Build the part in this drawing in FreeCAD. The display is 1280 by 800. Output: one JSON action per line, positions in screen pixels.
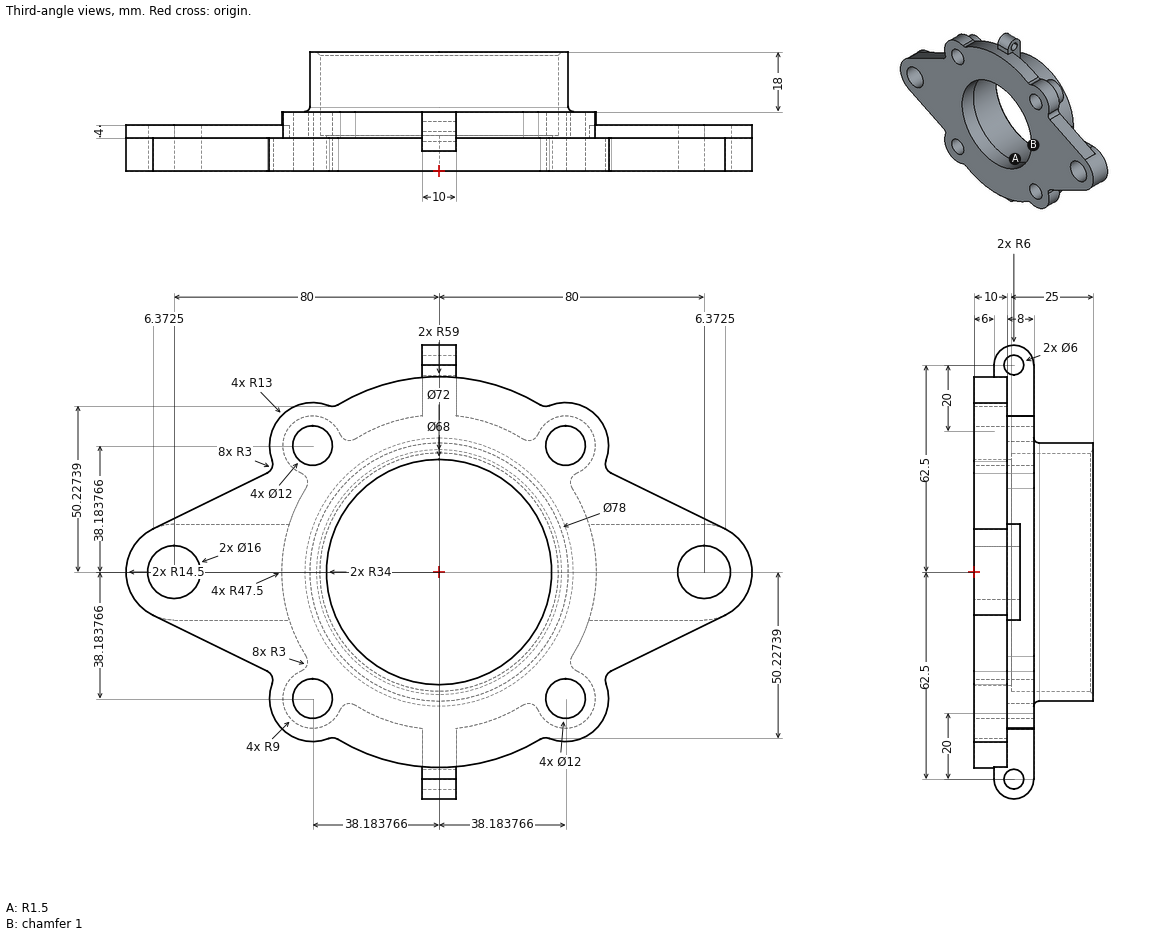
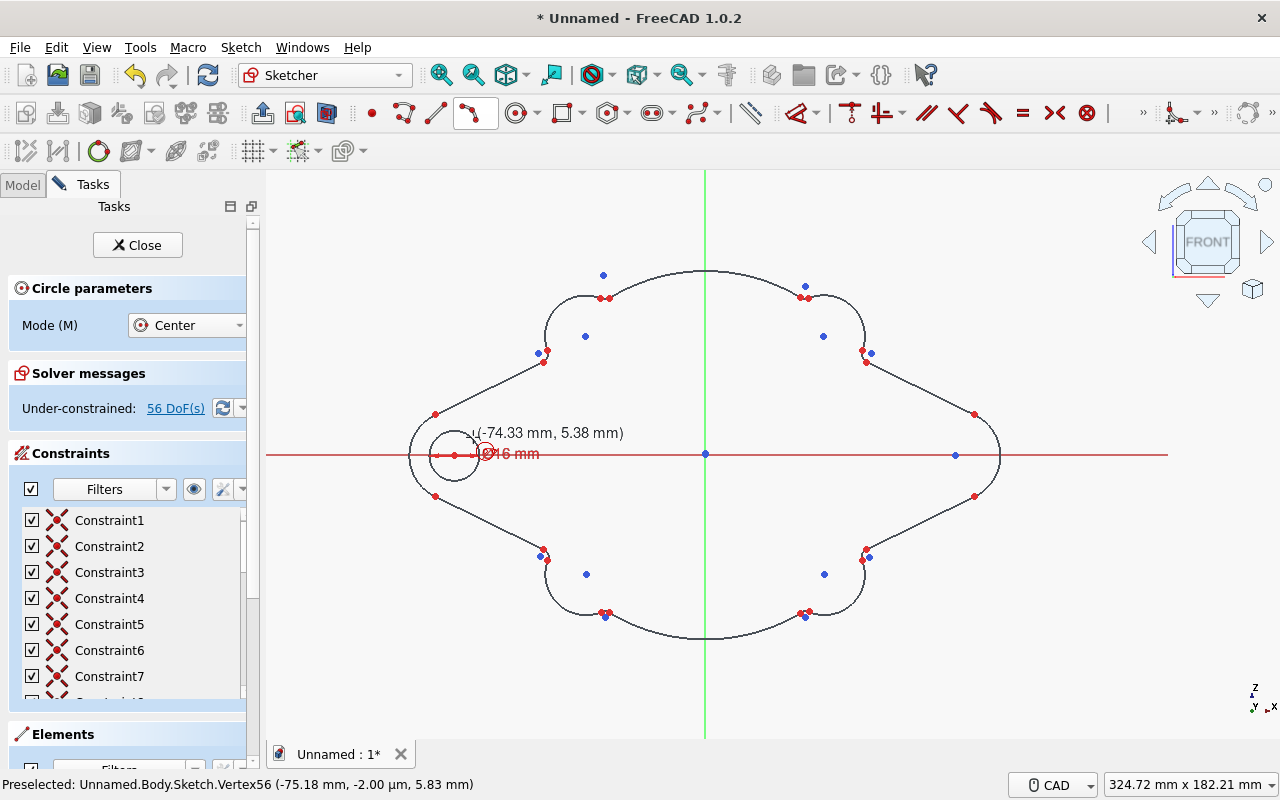
{"action": "left_click", "coordinate": [705, 455]}
{"action": "mouse_move", "coordinate": [780, 380]}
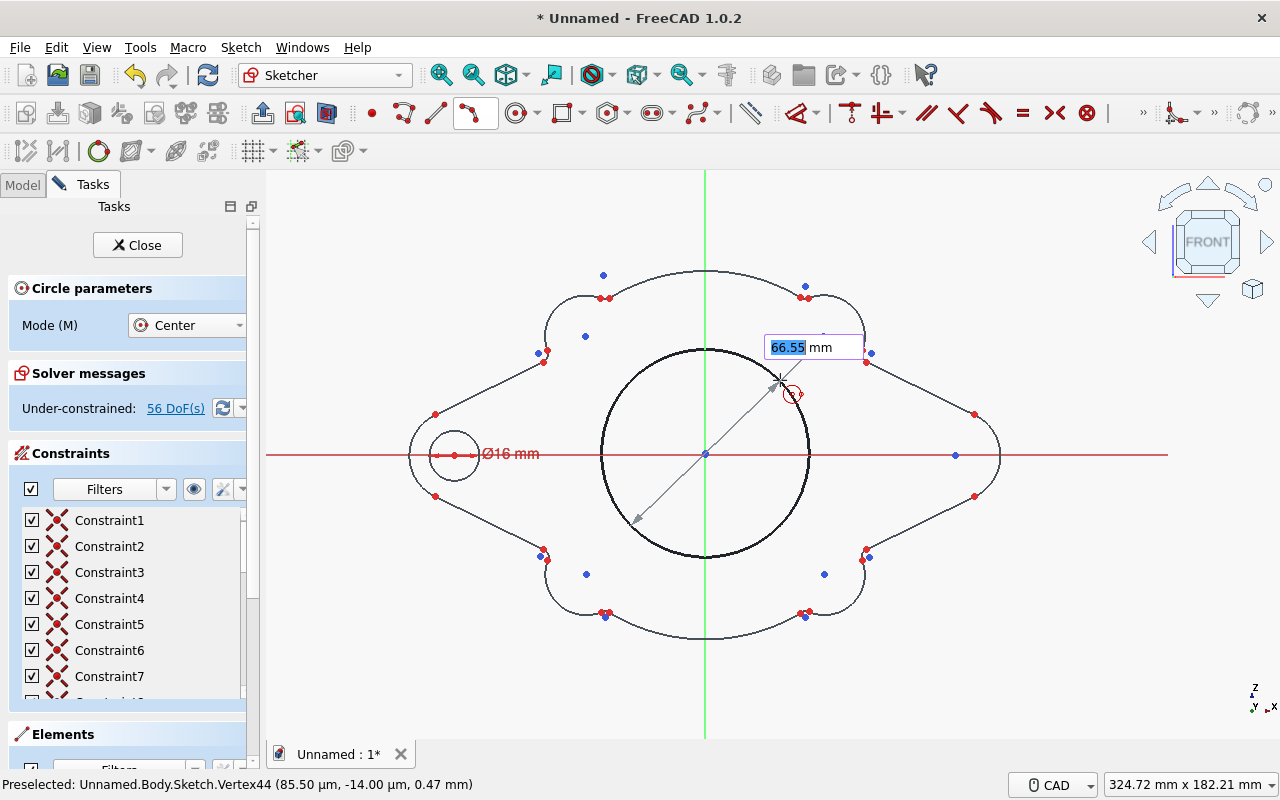
{"action": "type", "text": "68"}
{"action": "key", "text": "Return"}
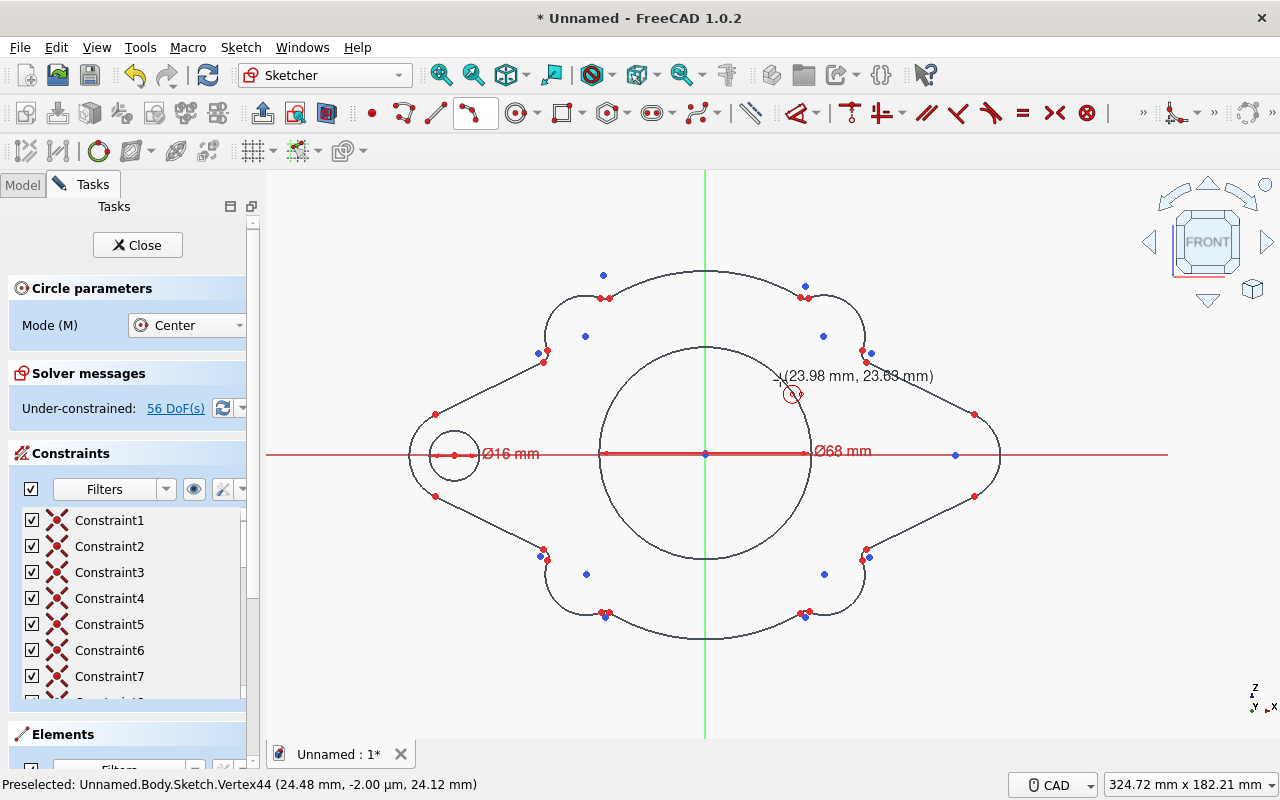
{"action": "left_click", "coordinate": [824, 574]}
{"action": "mouse_move", "coordinate": [838, 561]}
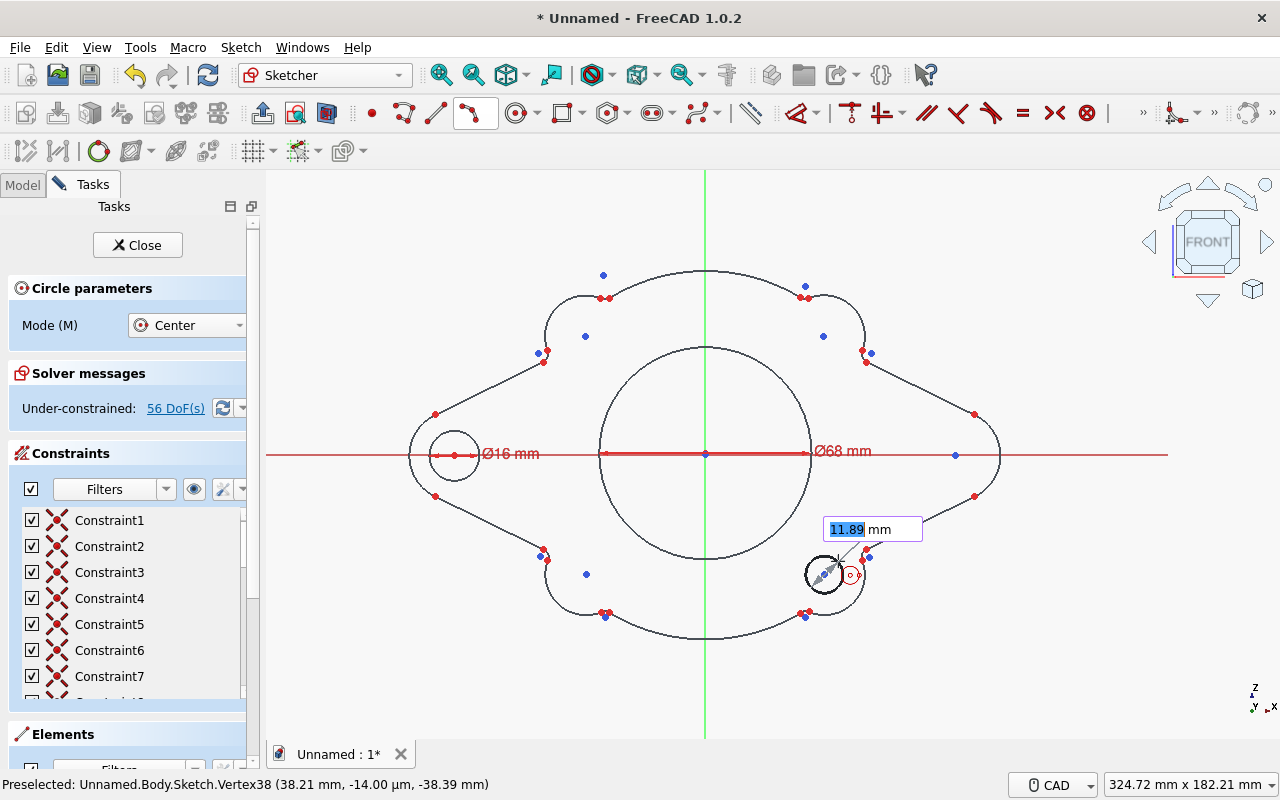
{"action": "type", "text": "12"}
{"action": "key", "text": "Return"}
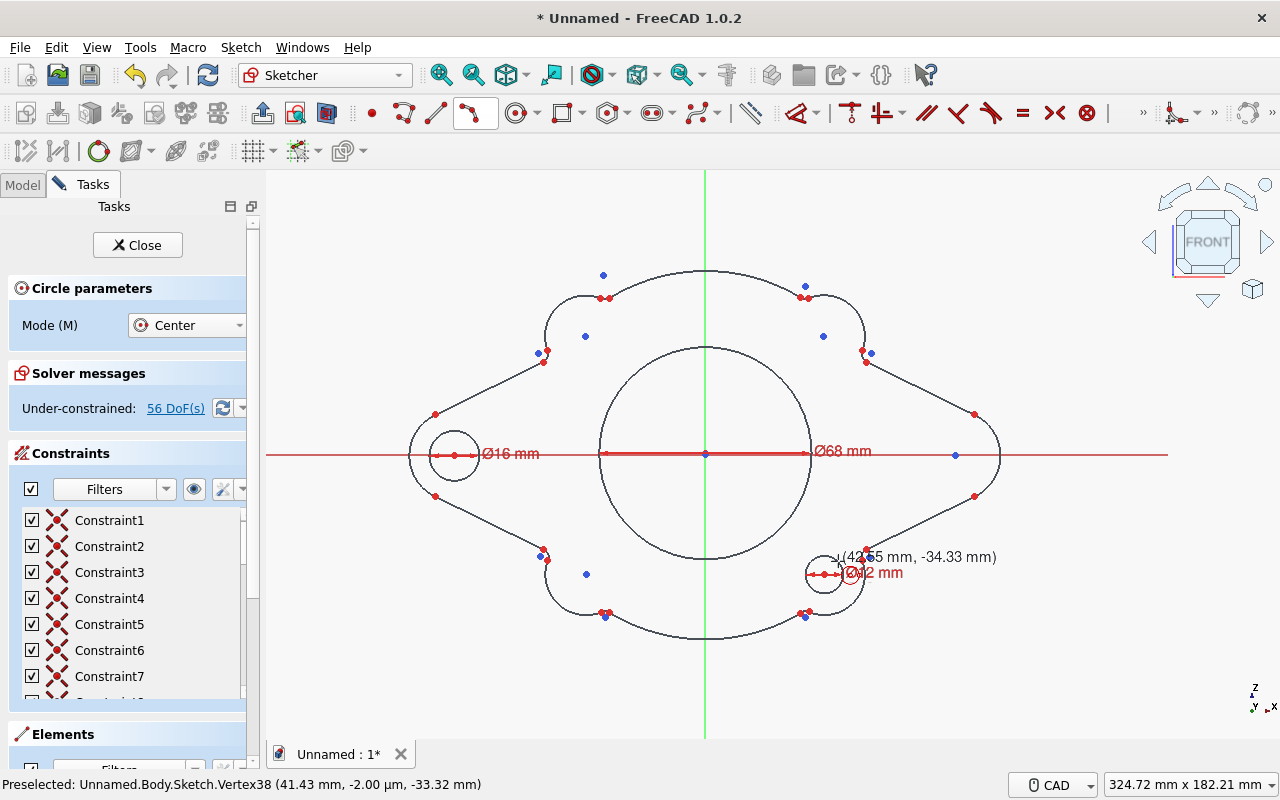
{"action": "left_click", "coordinate": [586, 574]}
{"action": "mouse_move", "coordinate": [599, 561]}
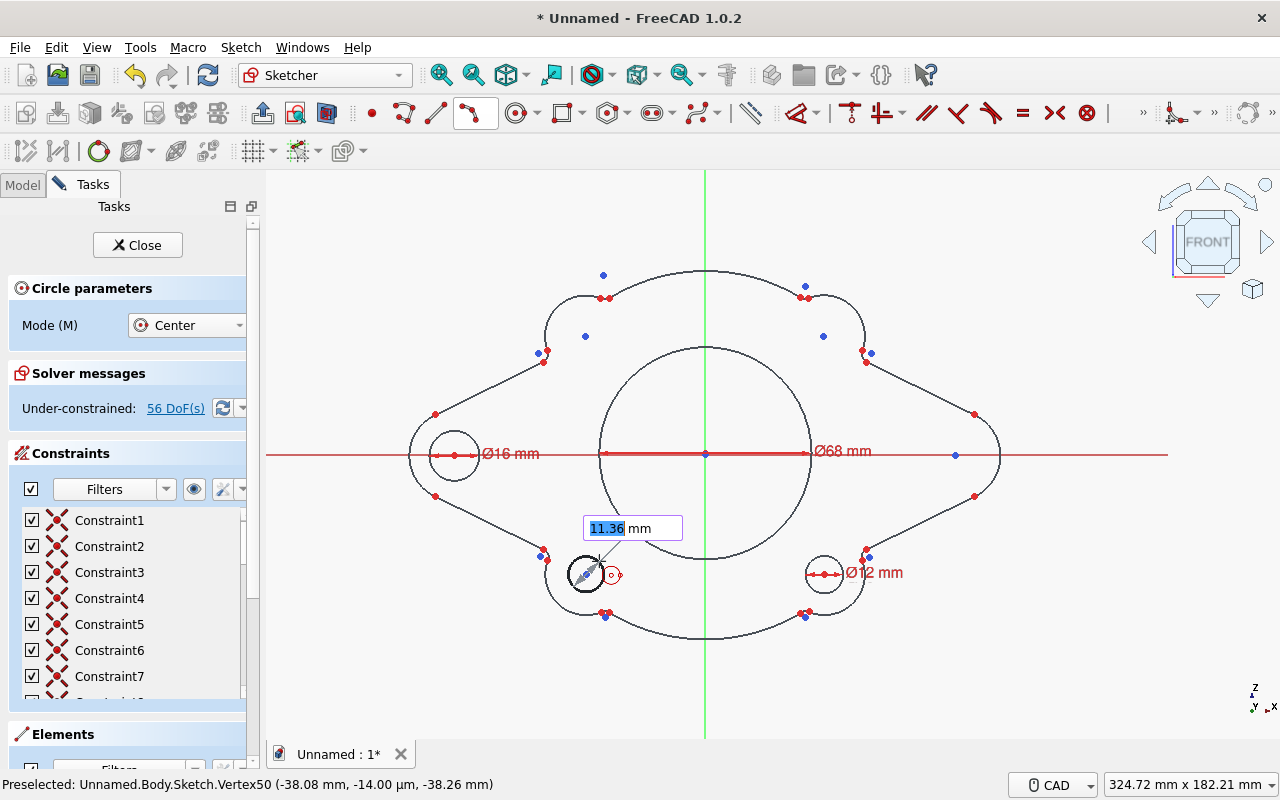
{"action": "type", "text": "12"}
{"action": "key", "text": "Return"}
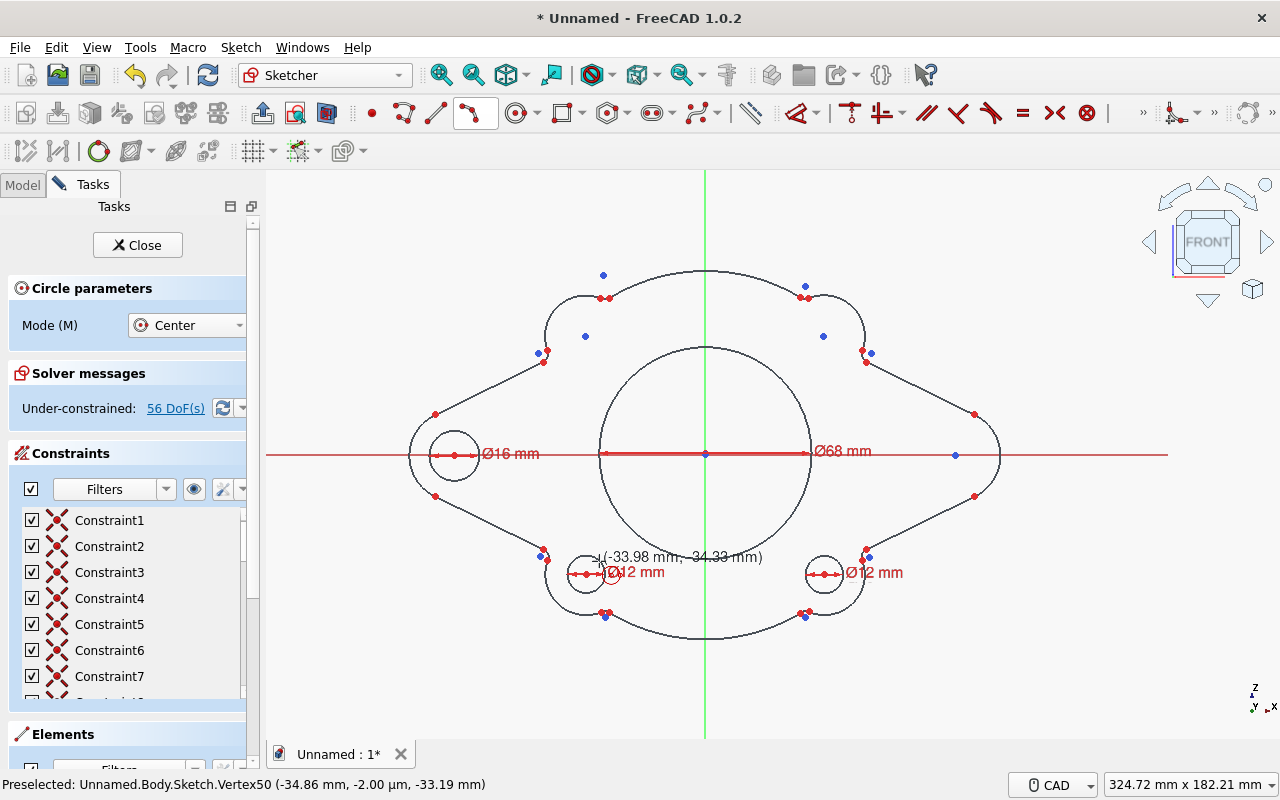
{"action": "left_click", "coordinate": [824, 336]}
{"action": "mouse_move", "coordinate": [838, 322]}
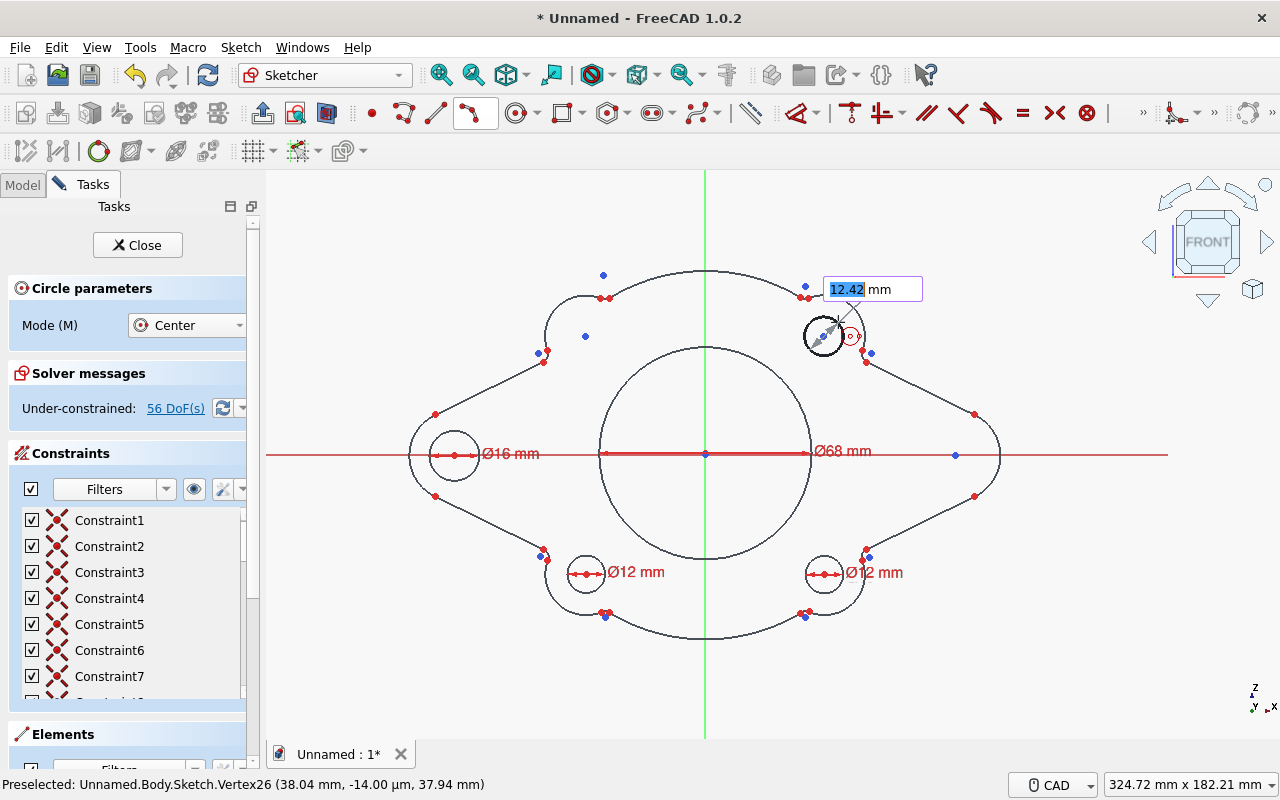
{"action": "type", "text": "12"}
{"action": "key", "text": "Return"}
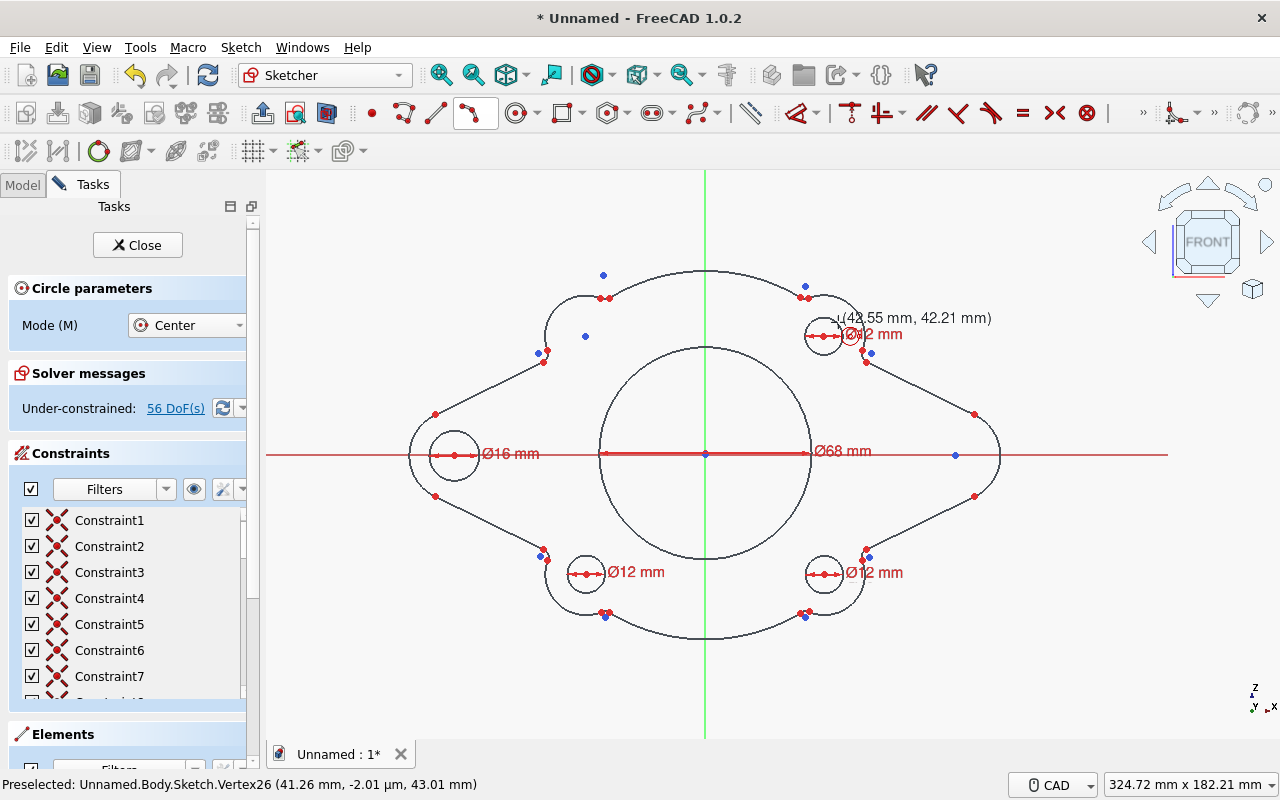
{"action": "left_click", "coordinate": [586, 336]}
{"action": "mouse_move", "coordinate": [599, 322]}